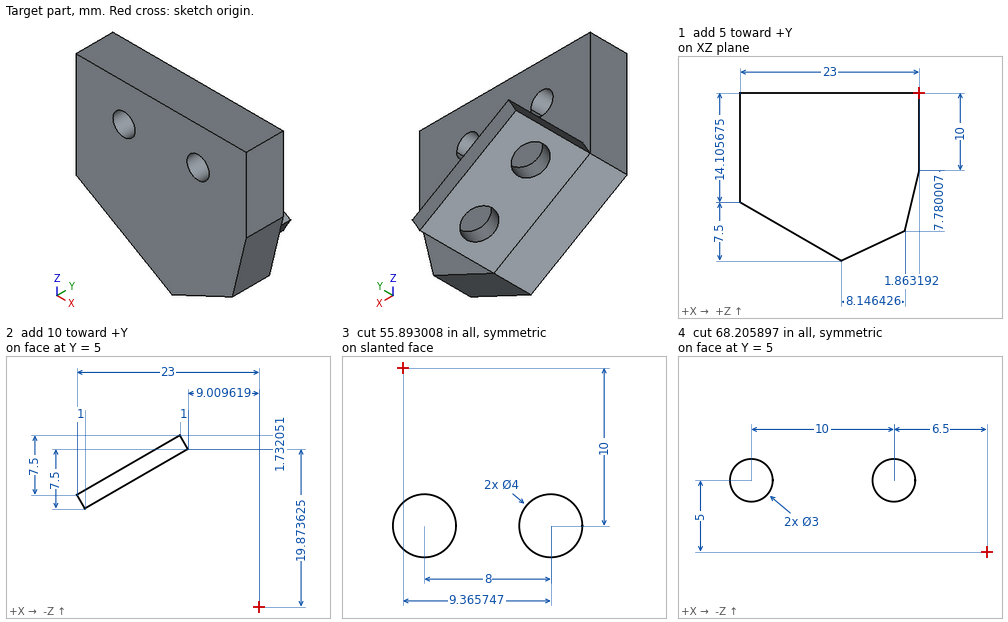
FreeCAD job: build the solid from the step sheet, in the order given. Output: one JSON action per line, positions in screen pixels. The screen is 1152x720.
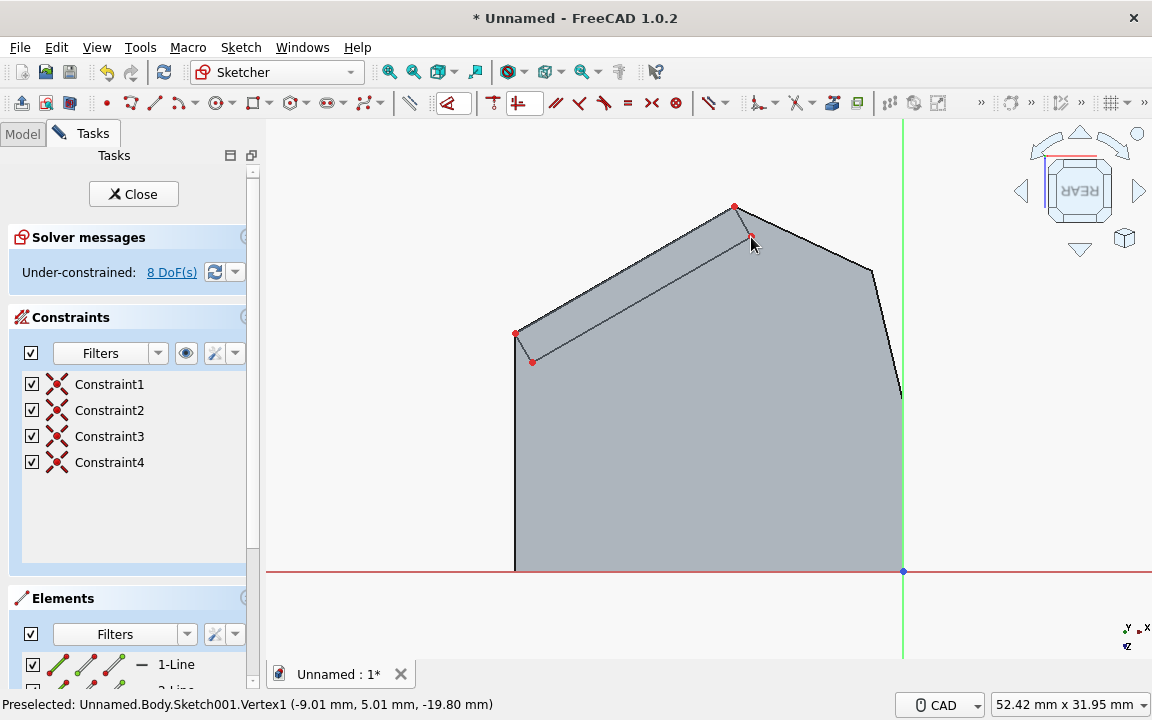
{"action": "scroll", "coordinate": [746, 228], "scroll_direction": "up", "scroll_amount": 5}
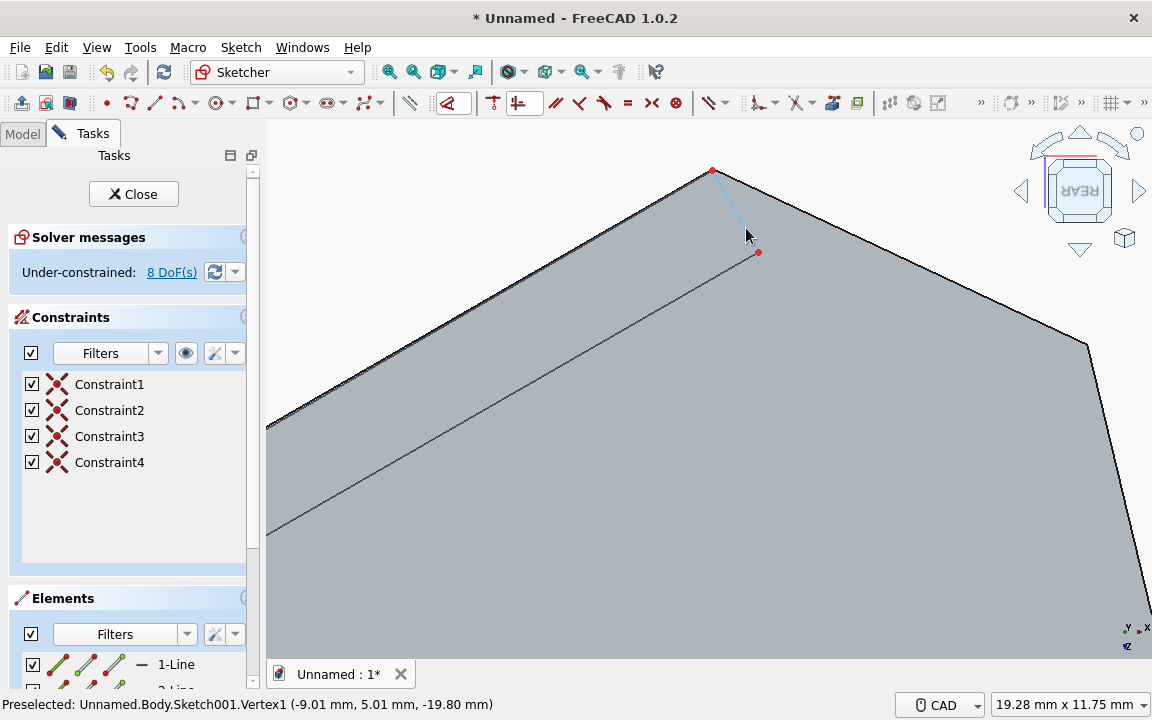
{"action": "left_click", "coordinate": [745, 228]}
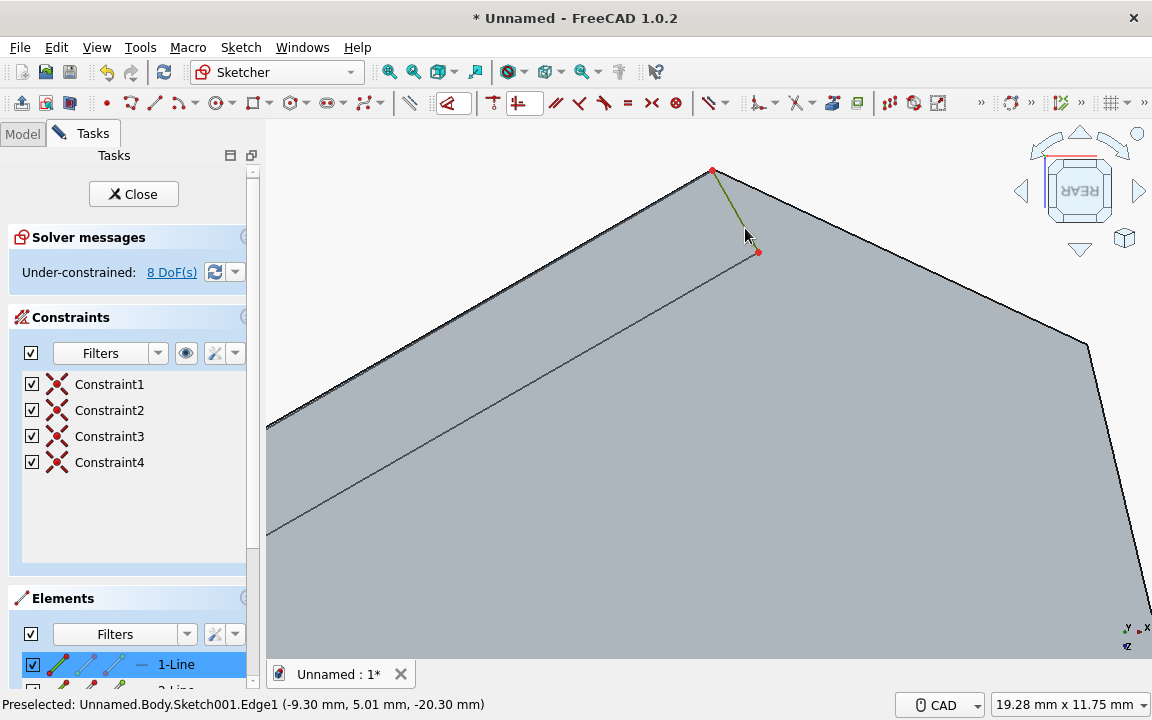
{"action": "left_click", "coordinate": [466, 104]}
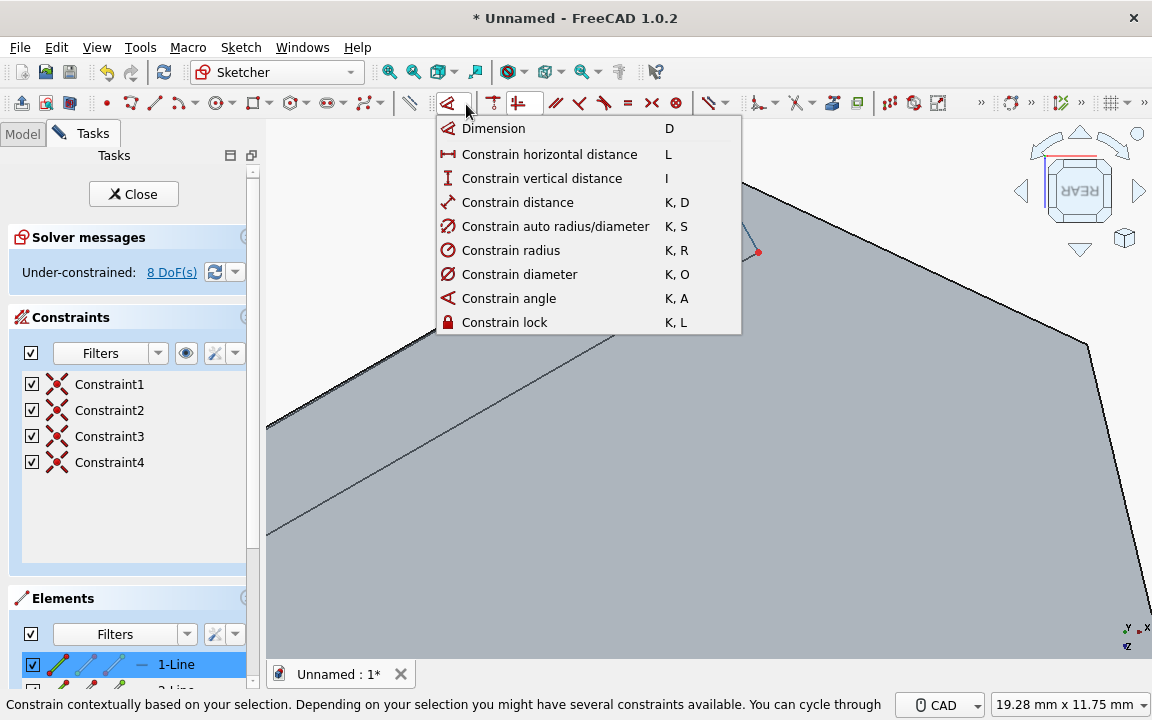
{"action": "left_click", "coordinate": [589, 154]}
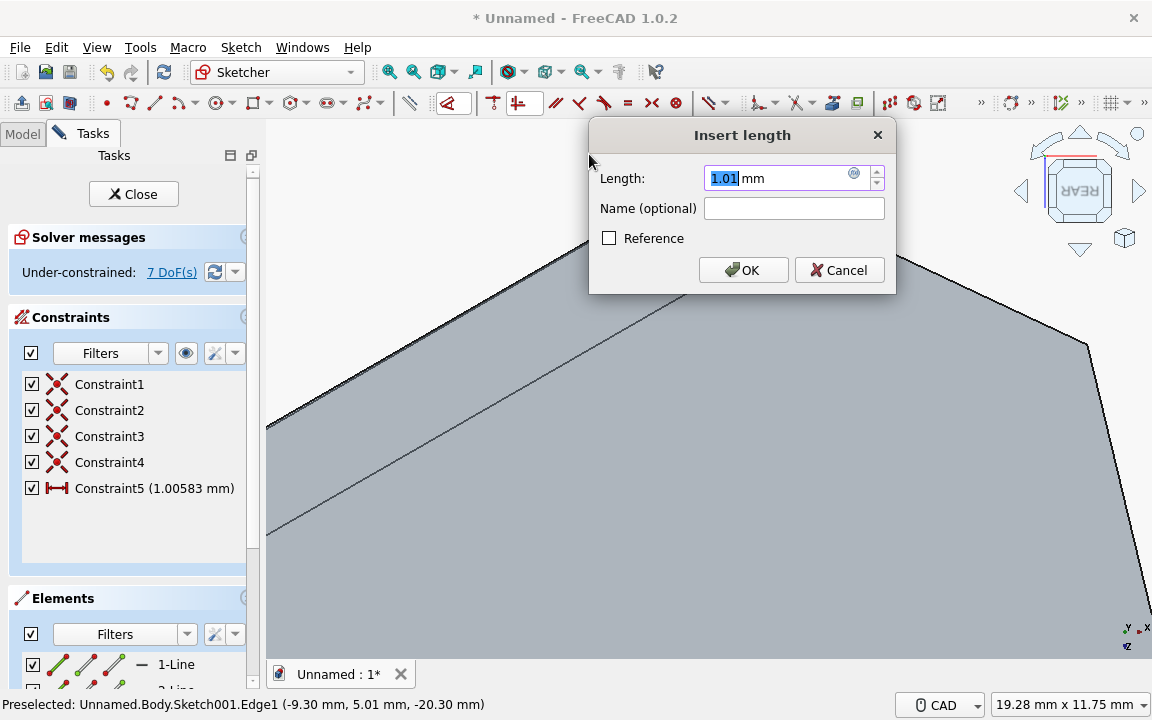
{"action": "type", "text": "1"}
{"action": "key", "text": "Return"}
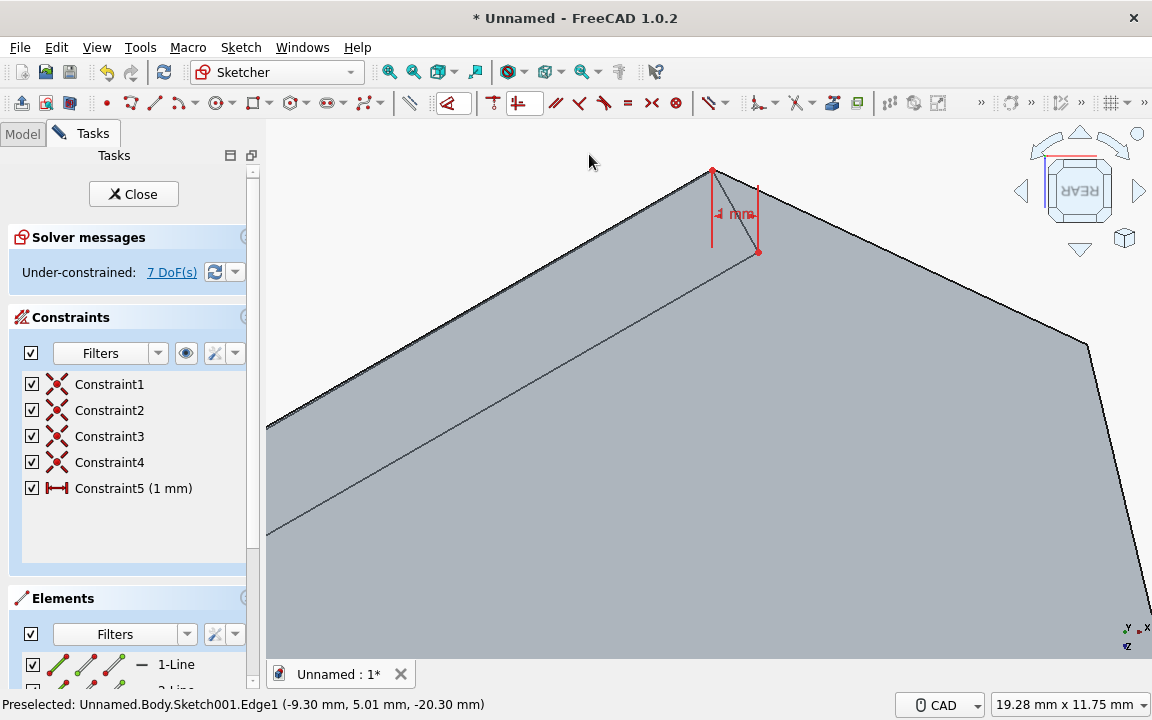
{"action": "scroll", "coordinate": [638, 228], "scroll_direction": "down", "scroll_amount": 5}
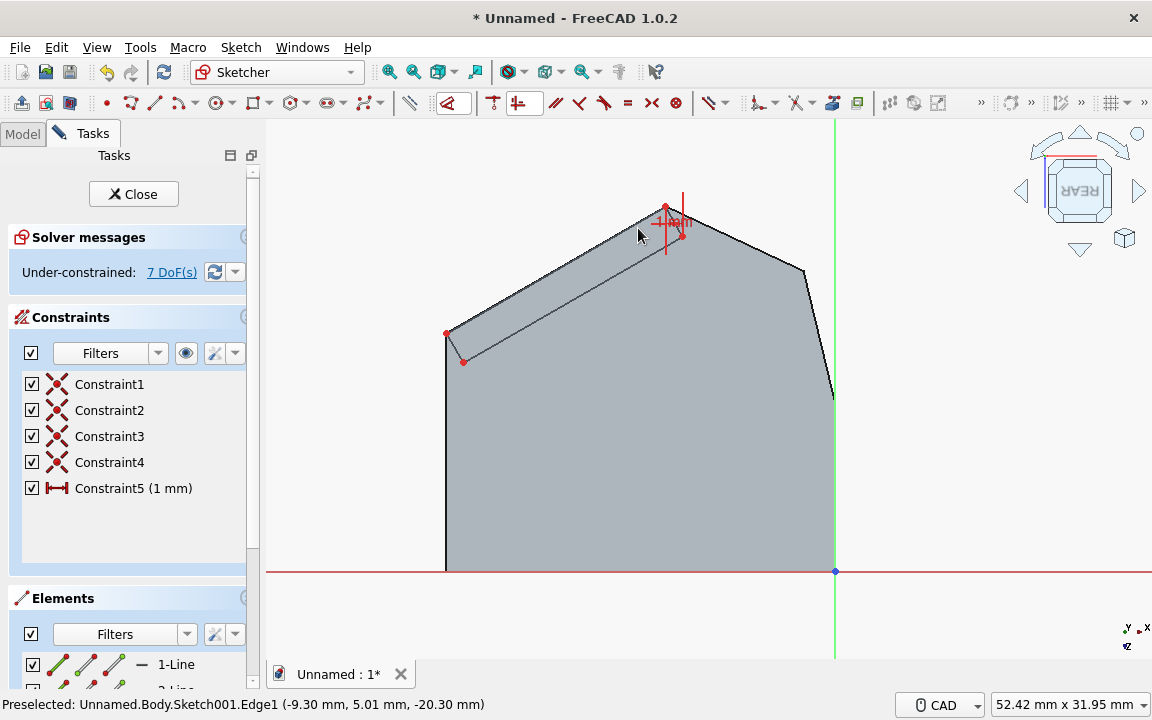
{"action": "scroll", "coordinate": [452, 343], "scroll_direction": "up", "scroll_amount": 5}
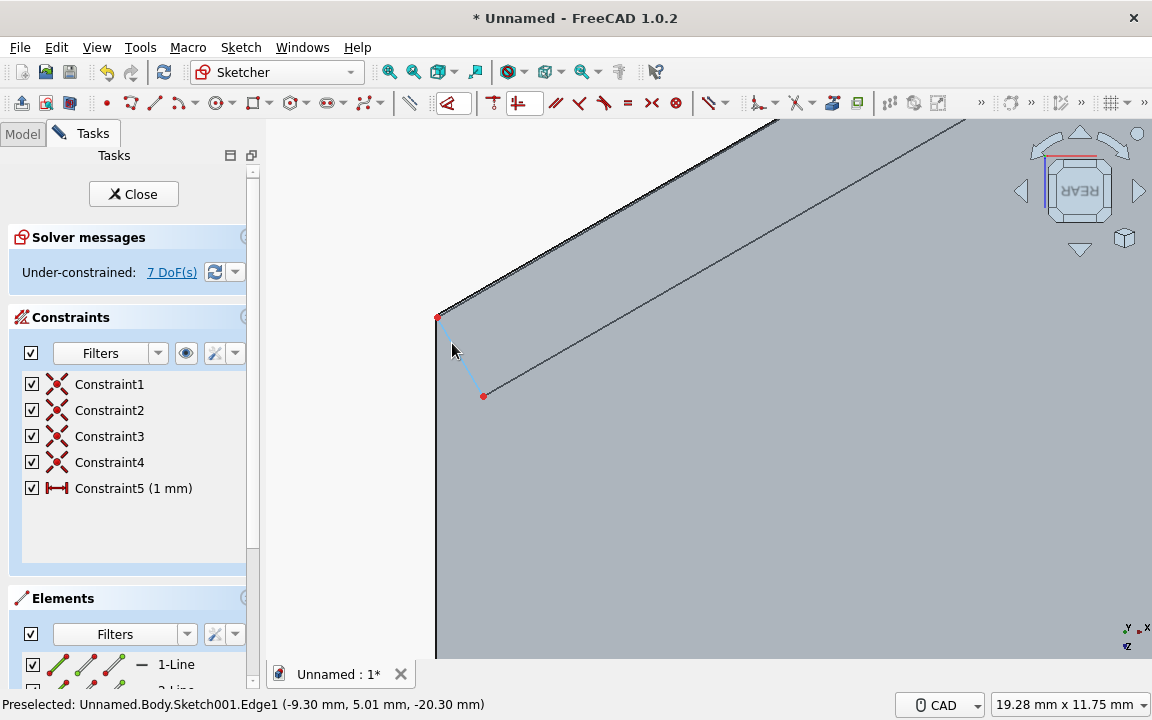
{"action": "left_click", "coordinate": [451, 341]}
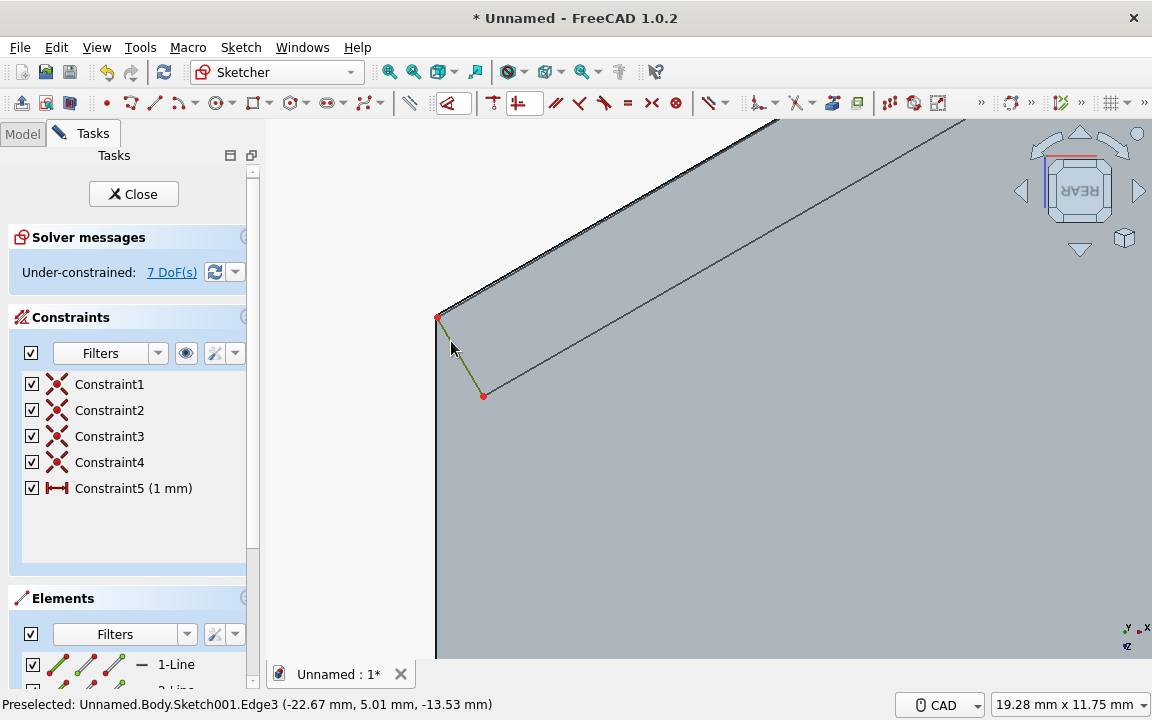
{"action": "left_click", "coordinate": [466, 104]}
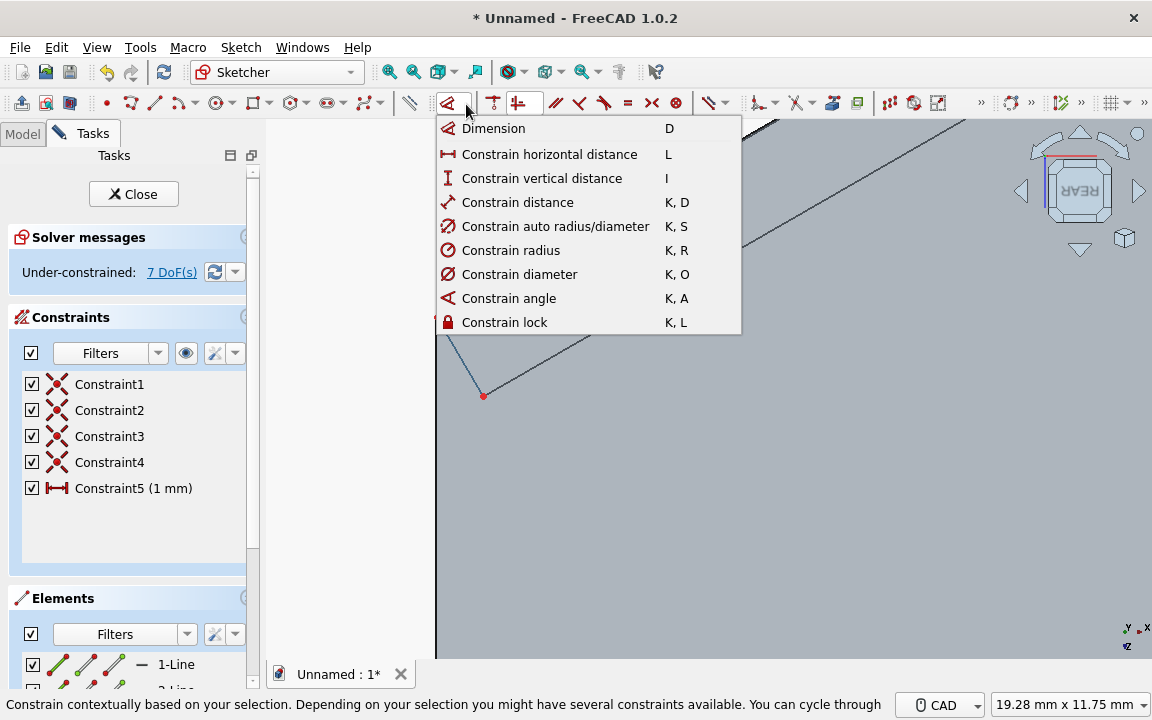
{"action": "left_click", "coordinate": [589, 154]}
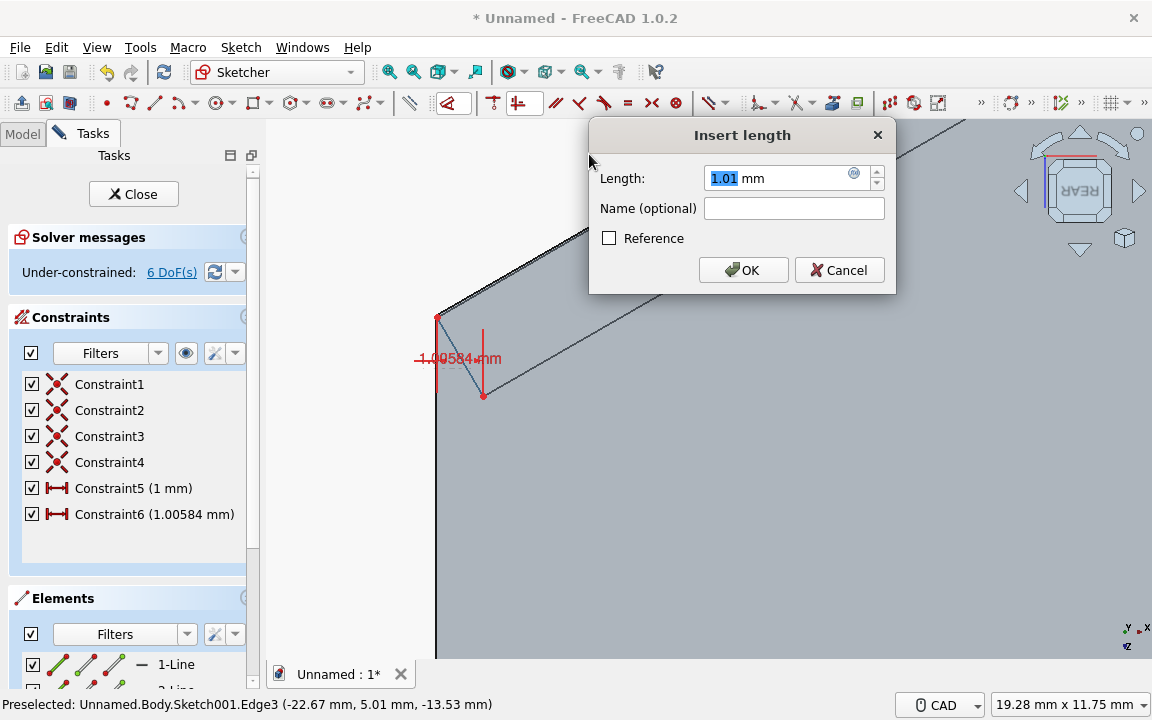
{"action": "type", "text": "1"}
{"action": "key", "text": "Return"}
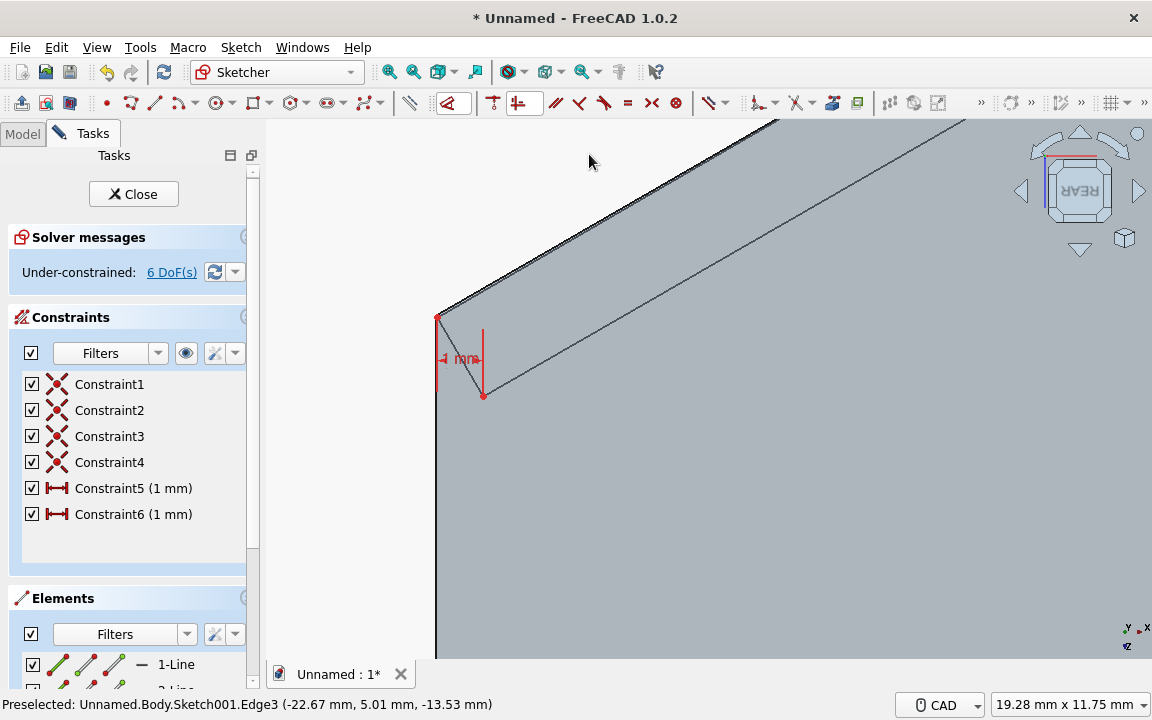
{"action": "left_click", "coordinate": [437, 318]}